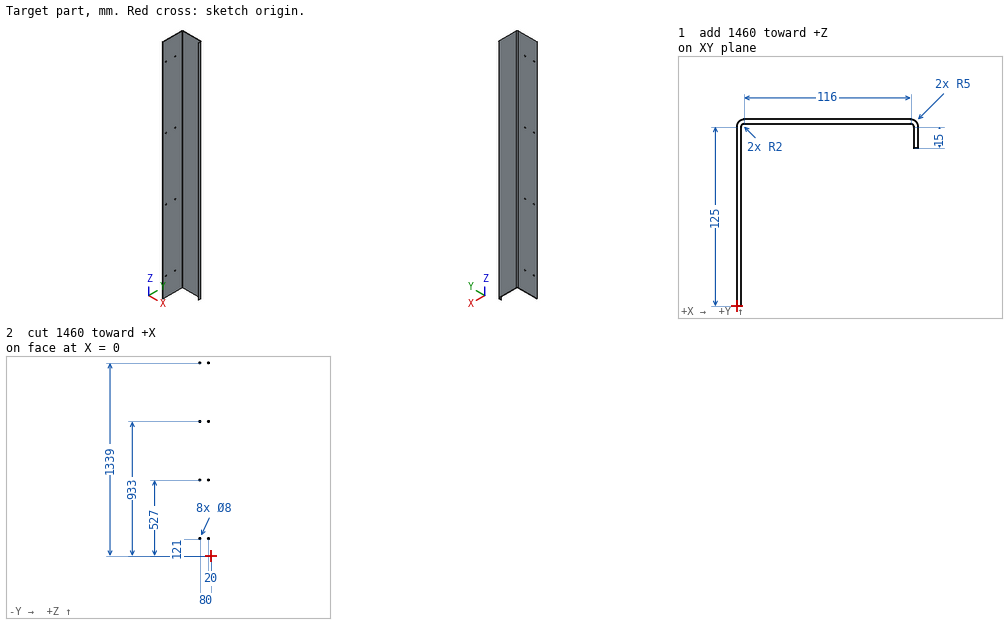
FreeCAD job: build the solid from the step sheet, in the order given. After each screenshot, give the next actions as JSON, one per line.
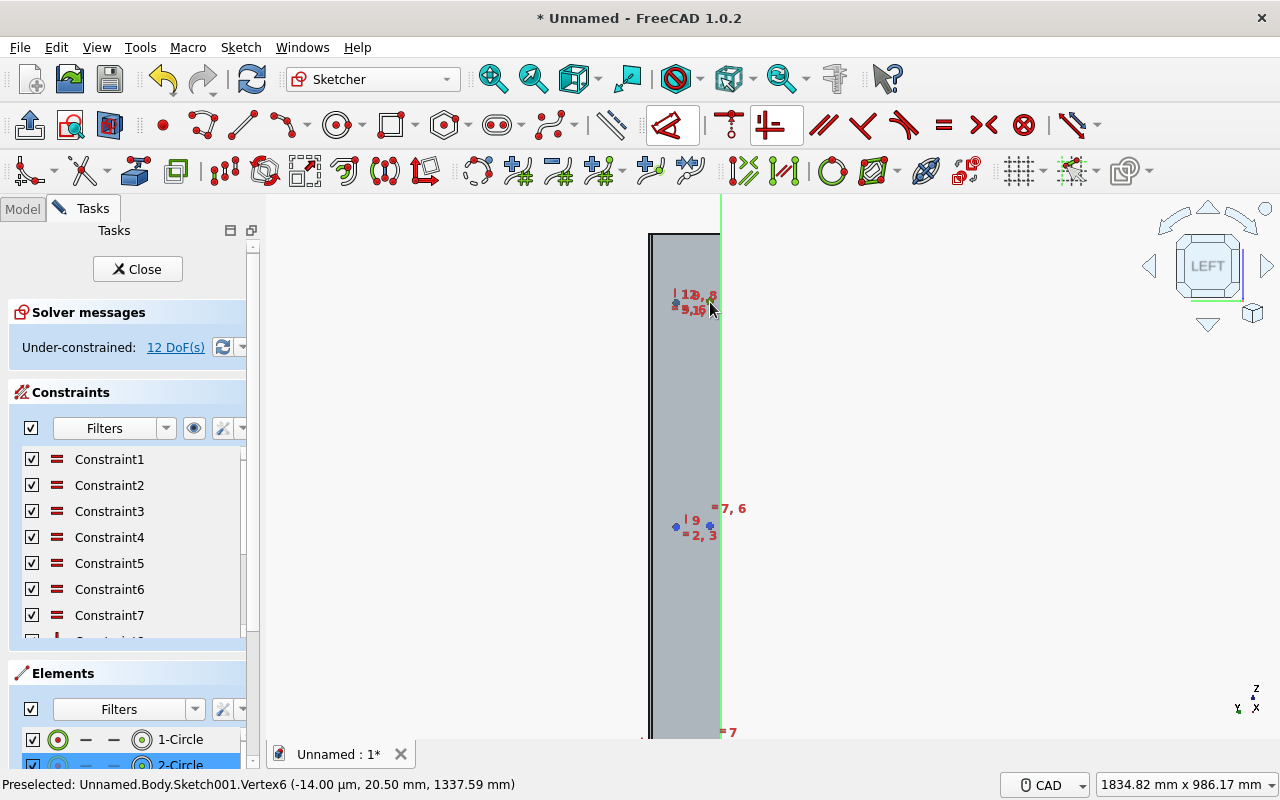
{"action": "key", "text": "h"}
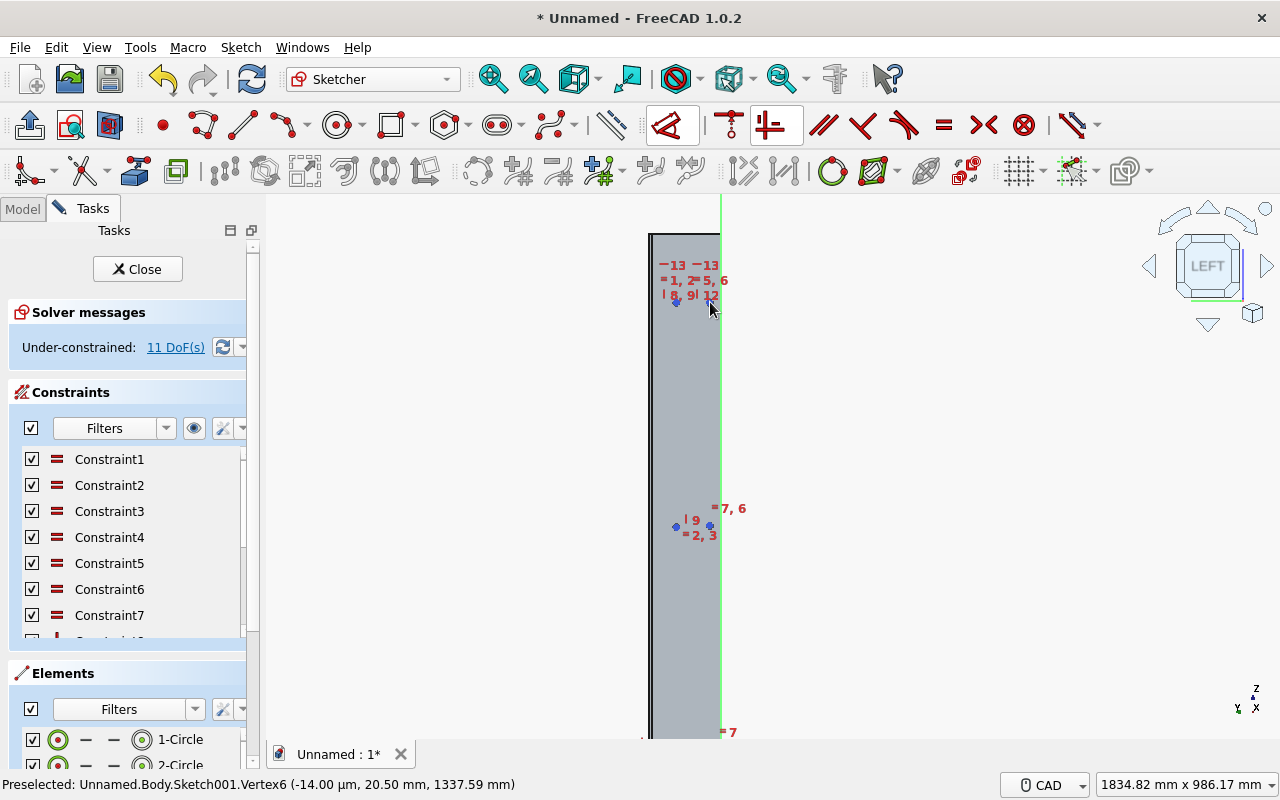
{"action": "left_click", "coordinate": [710, 303]}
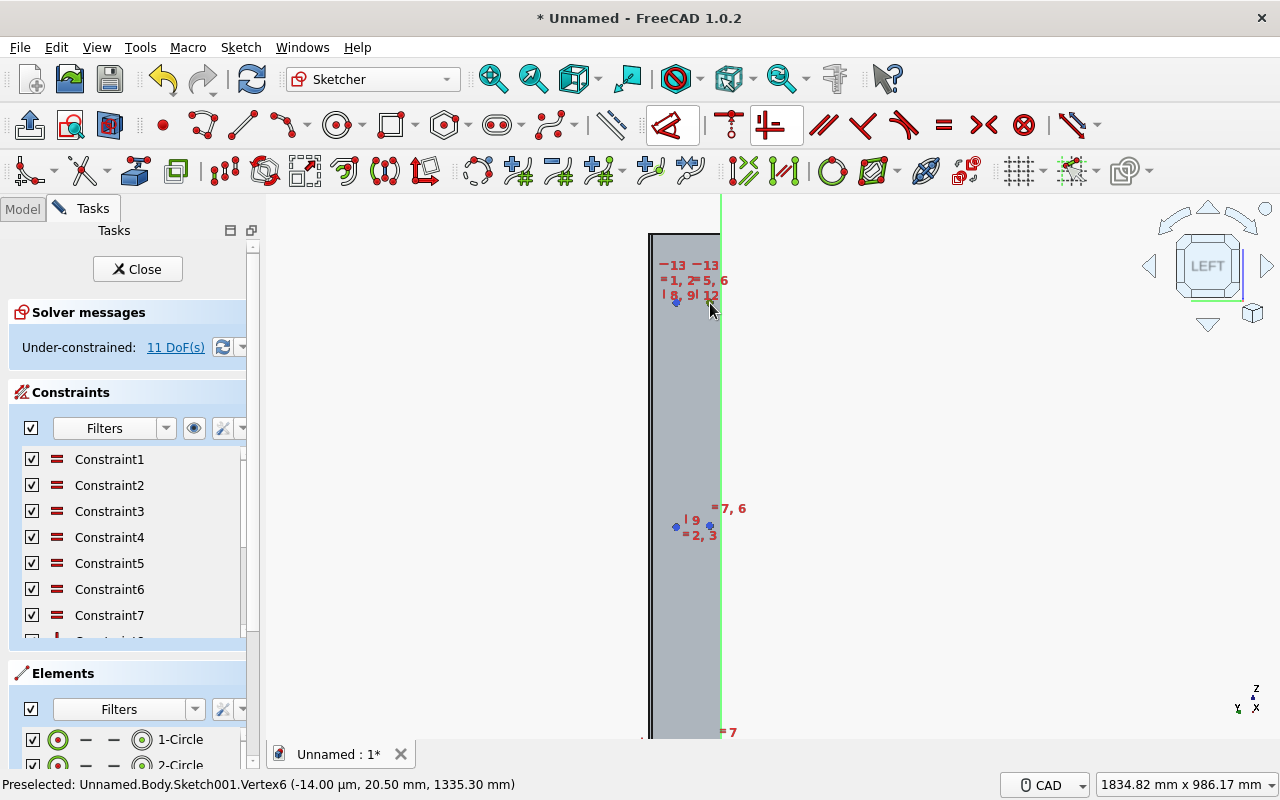
{"action": "scroll", "coordinate": [710, 526], "scroll_direction": "up", "scroll_amount": 4}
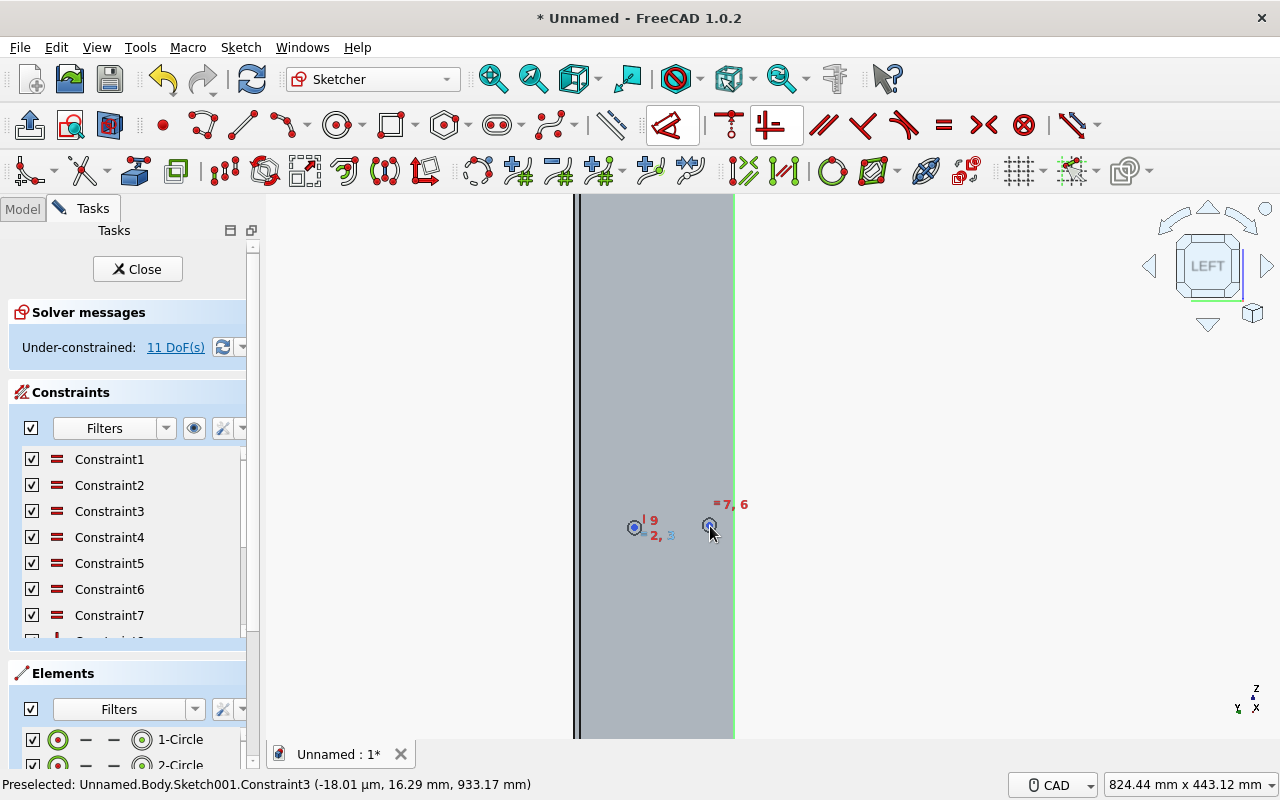
{"action": "left_click", "coordinate": [709, 525]}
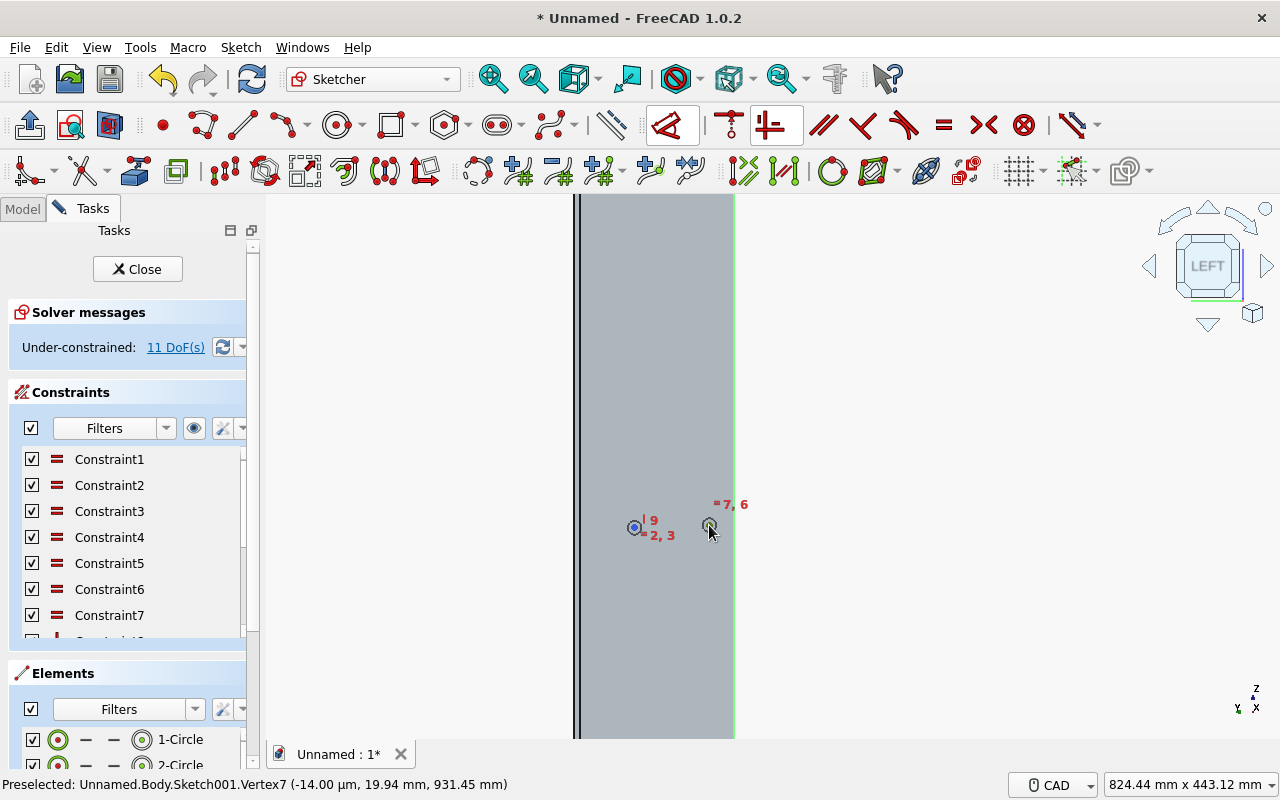
{"action": "key", "text": "v"}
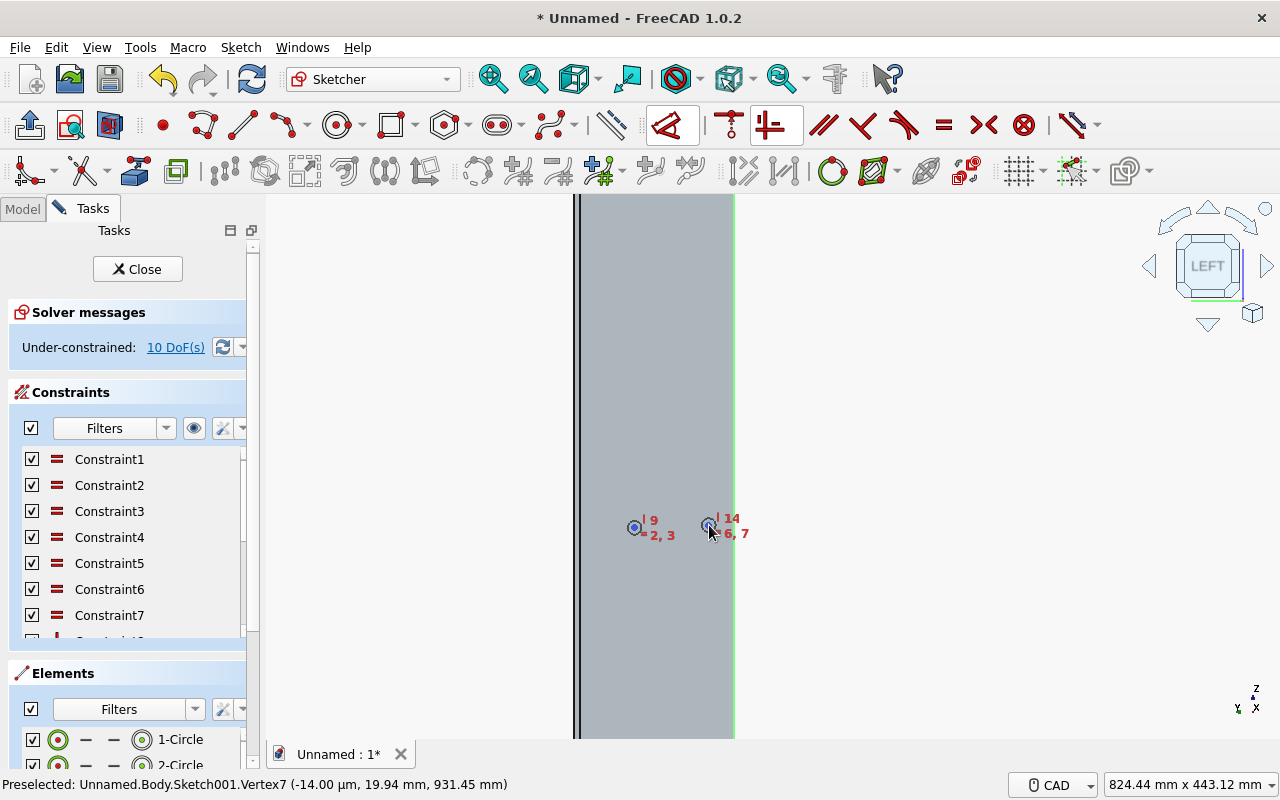
{"action": "scroll", "coordinate": [710, 371], "scroll_direction": "down", "scroll_amount": 8}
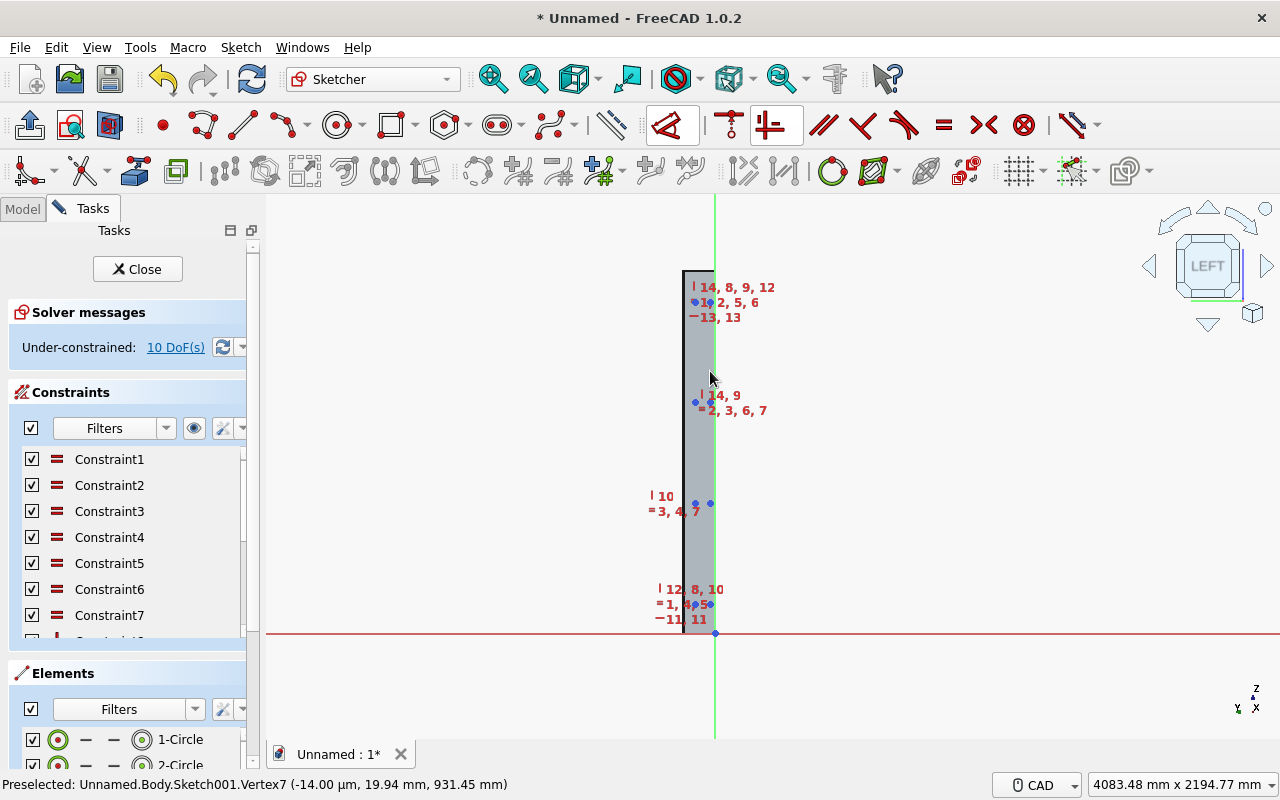
{"action": "left_click", "coordinate": [695, 403]}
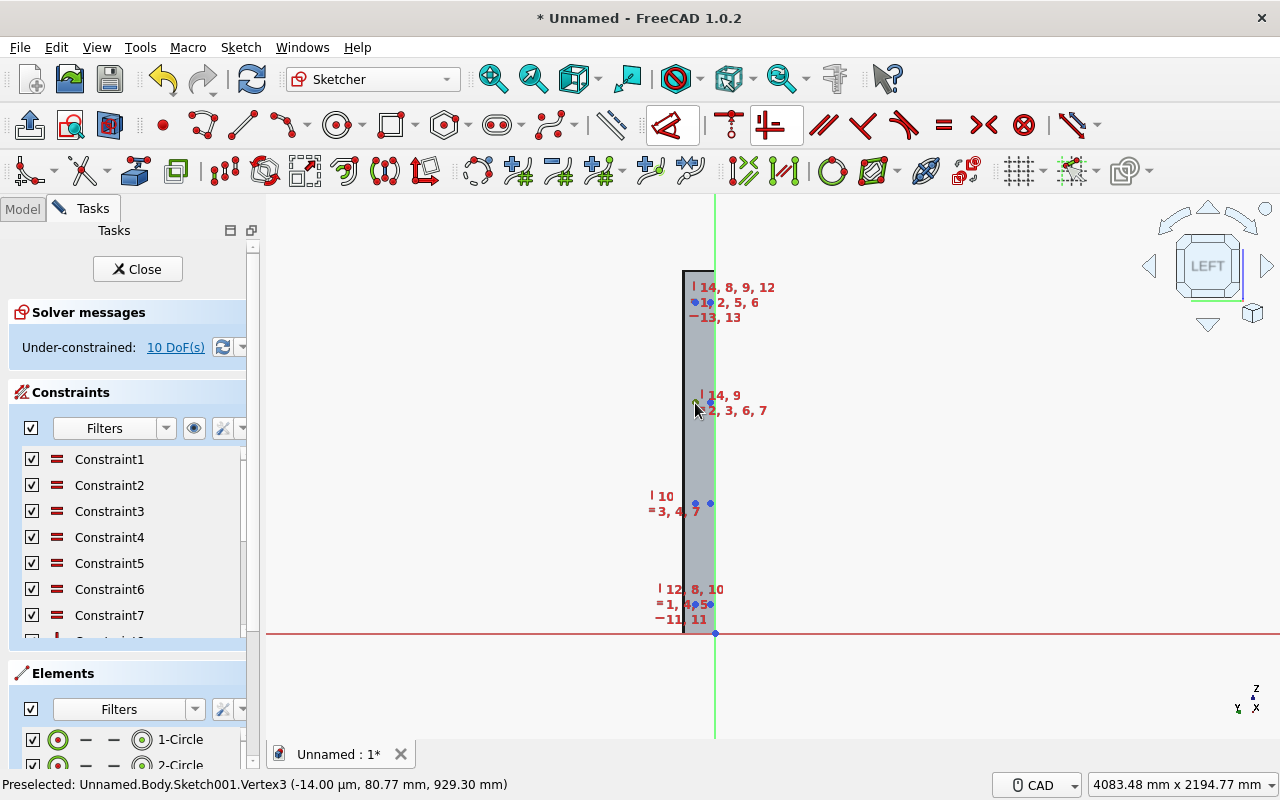
{"action": "scroll", "coordinate": [710, 402], "scroll_direction": "up", "scroll_amount": 4}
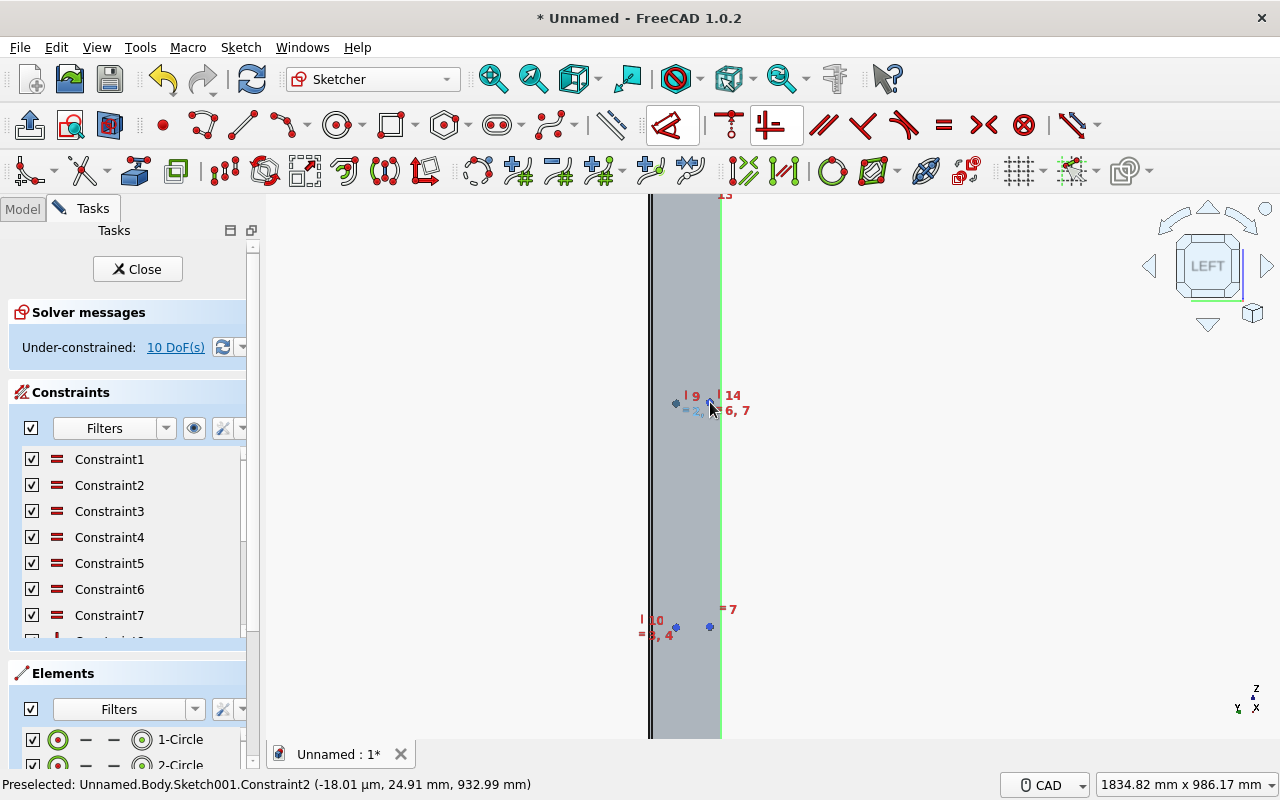
{"action": "scroll", "coordinate": [710, 402], "scroll_direction": "up", "scroll_amount": 4}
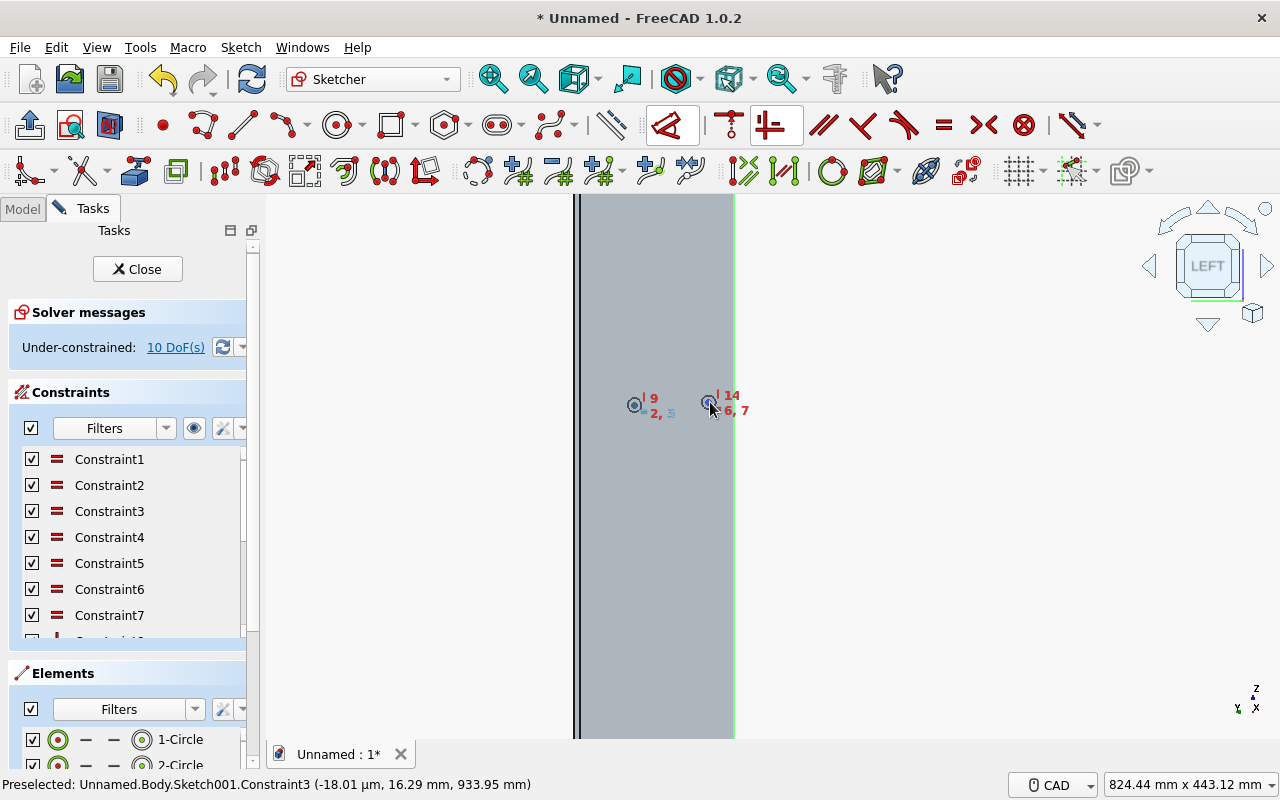
{"action": "left_click", "coordinate": [709, 402]}